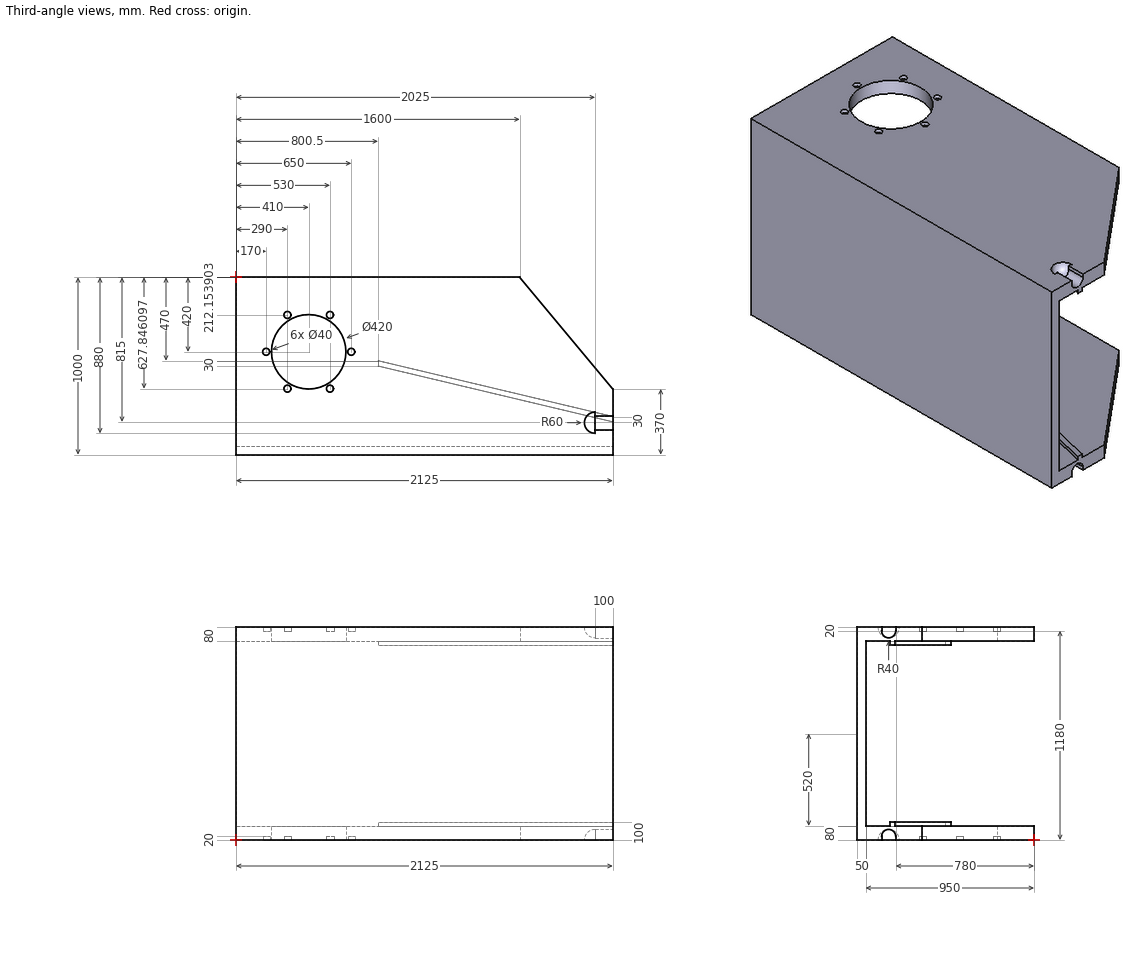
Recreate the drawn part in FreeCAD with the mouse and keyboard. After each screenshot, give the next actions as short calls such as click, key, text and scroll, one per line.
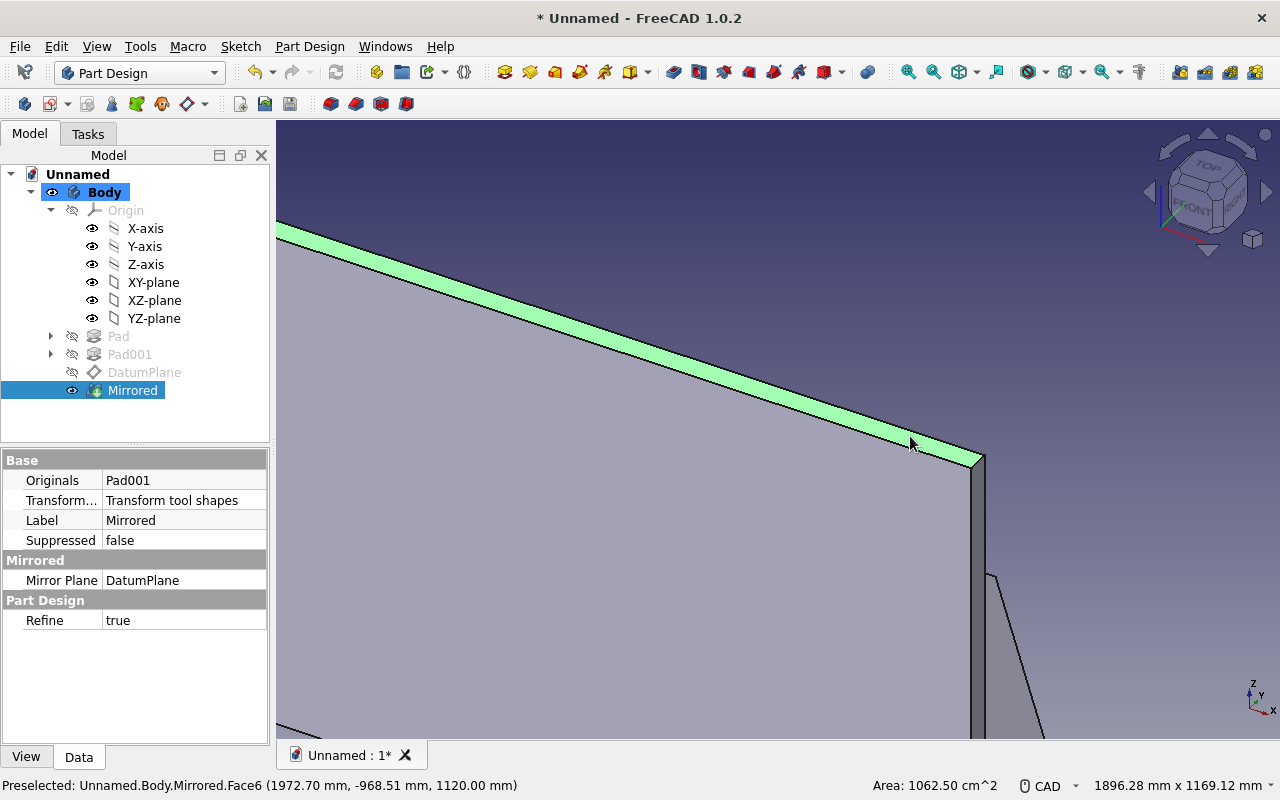
click(50, 104)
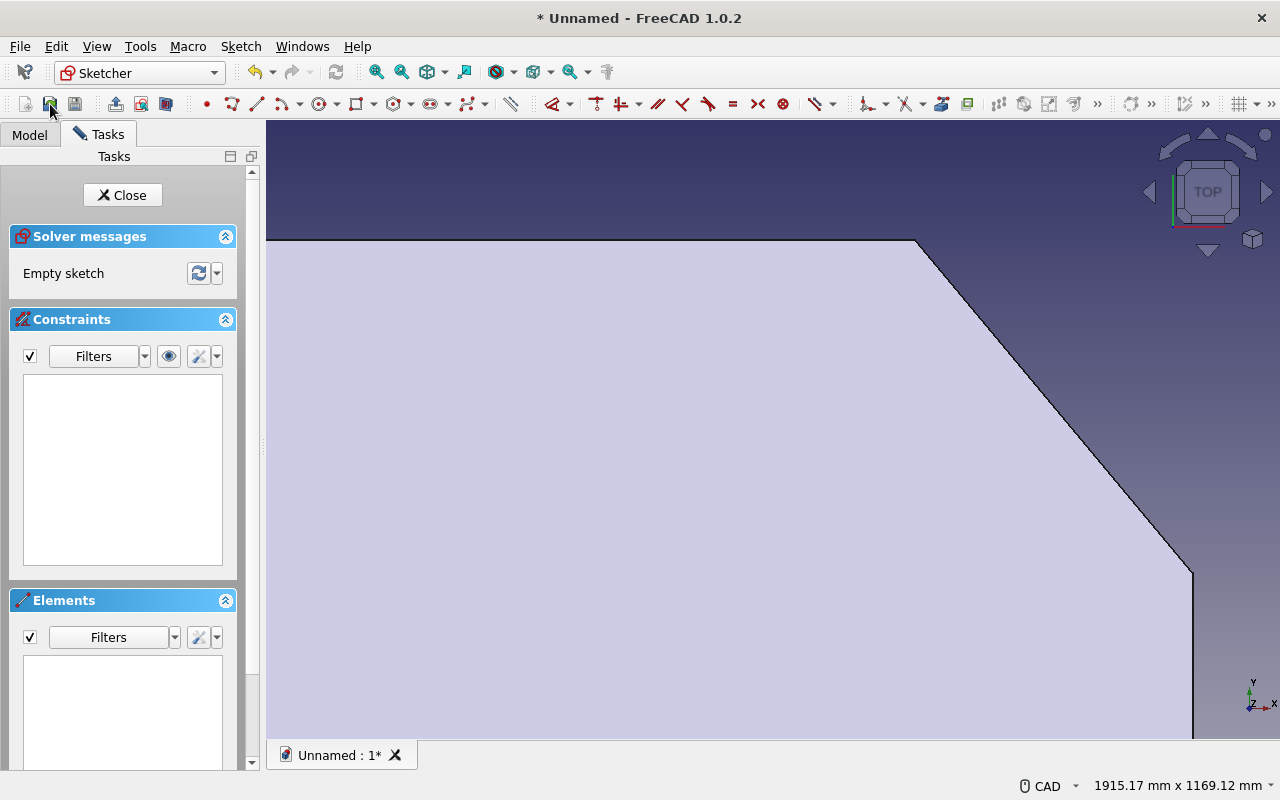
scroll(795, 338, down, 3)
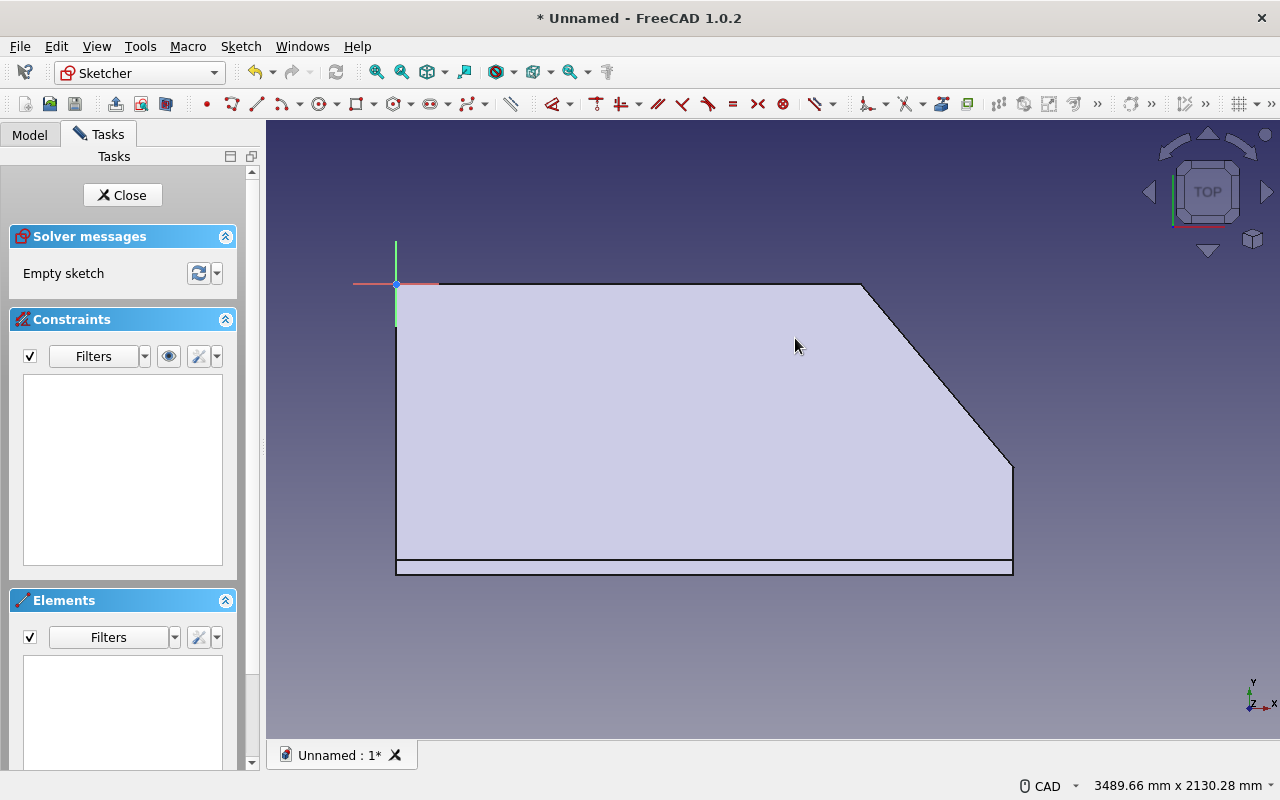
key(g)
key(m)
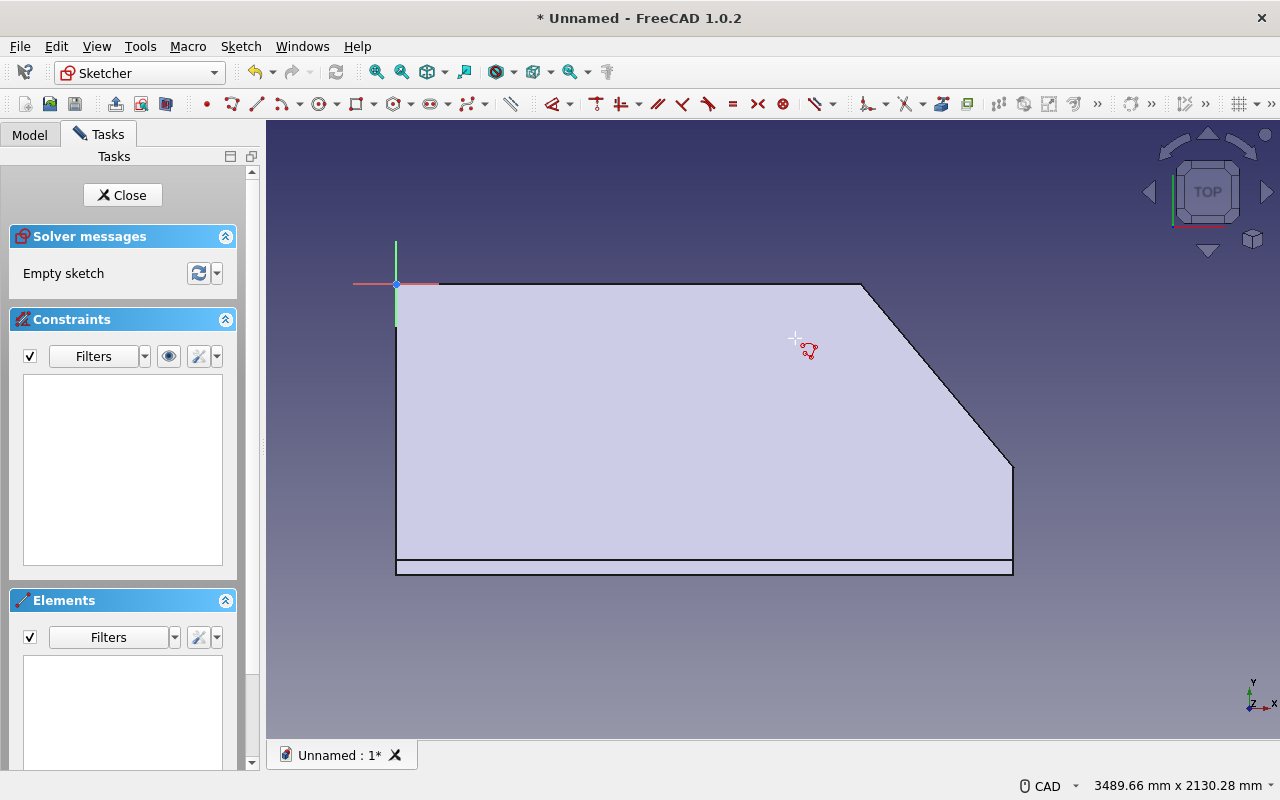
click(396, 284)
click(405, 575)
click(1013, 575)
click(1013, 467)
click(861, 293)
click(396, 284)
key(Escape)
key(Escape)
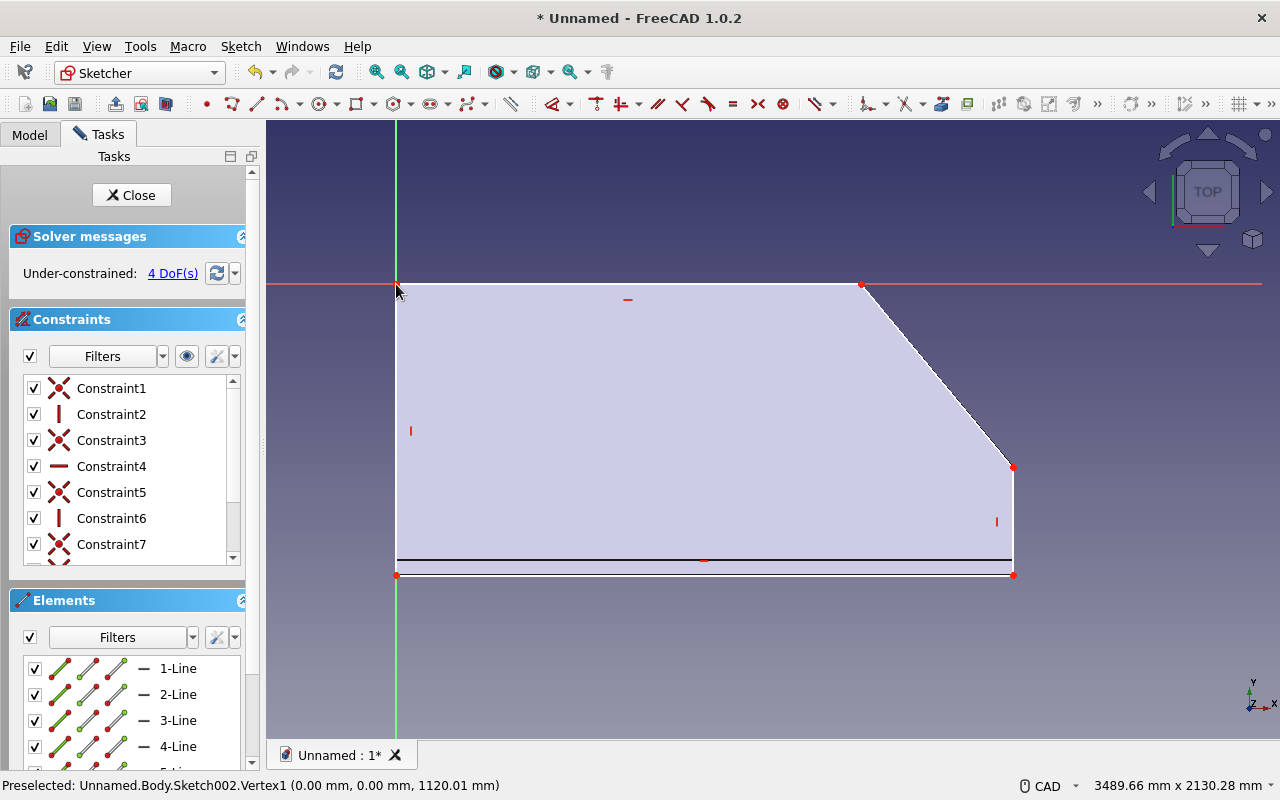
key(d)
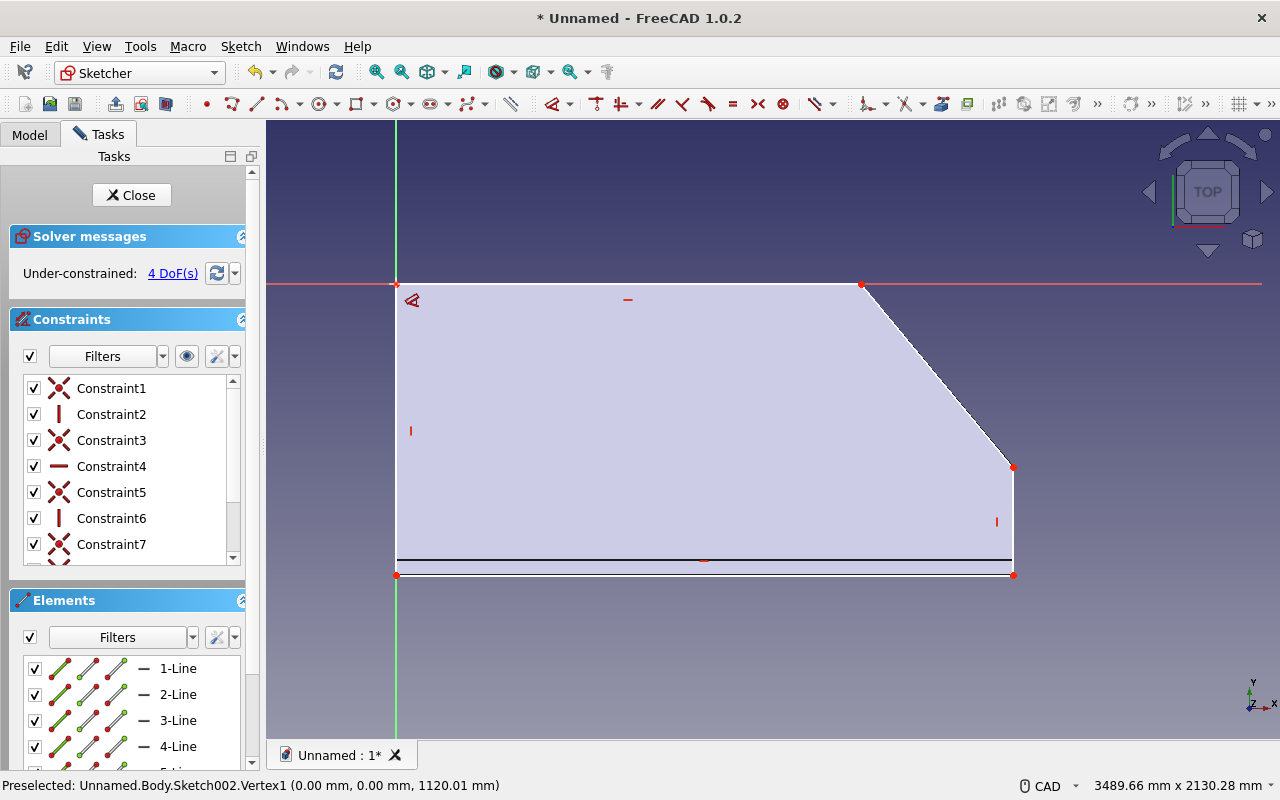
click(1013, 544)
click(1047, 522)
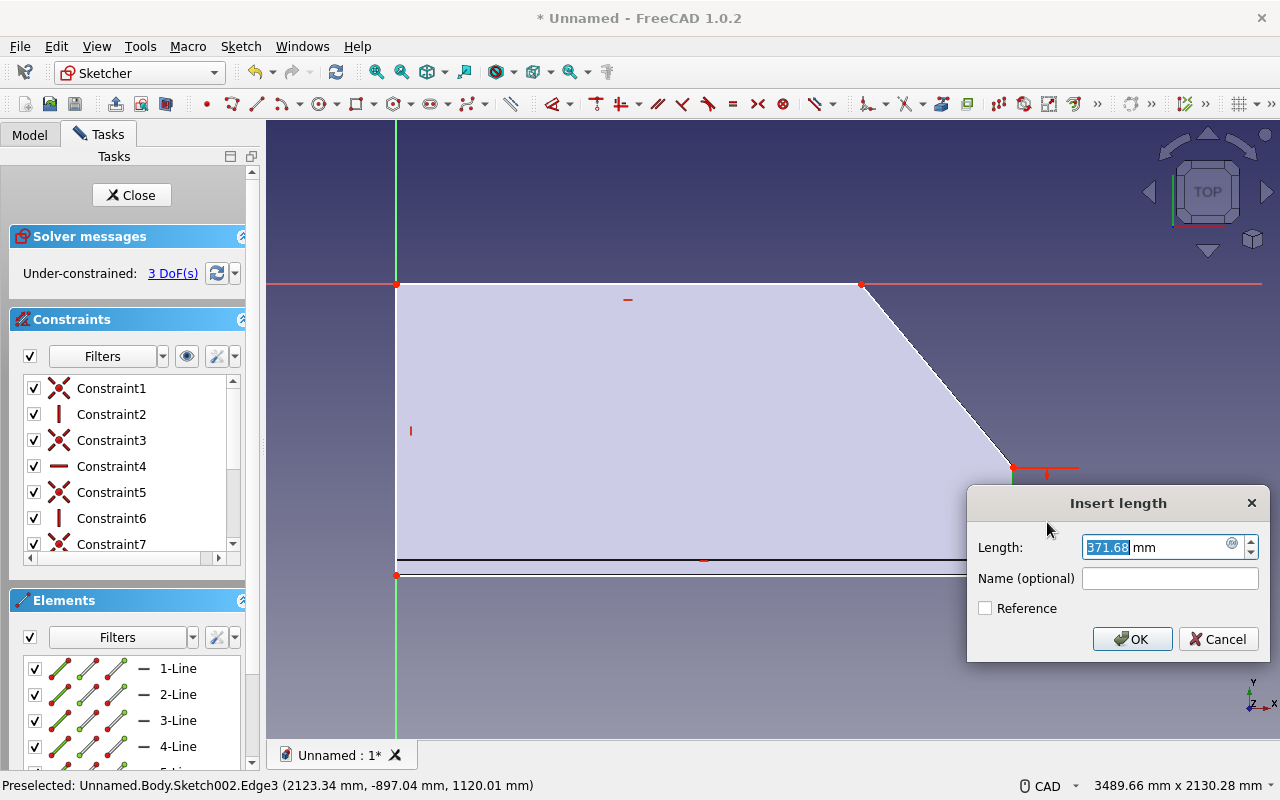
text(370)
key(Return)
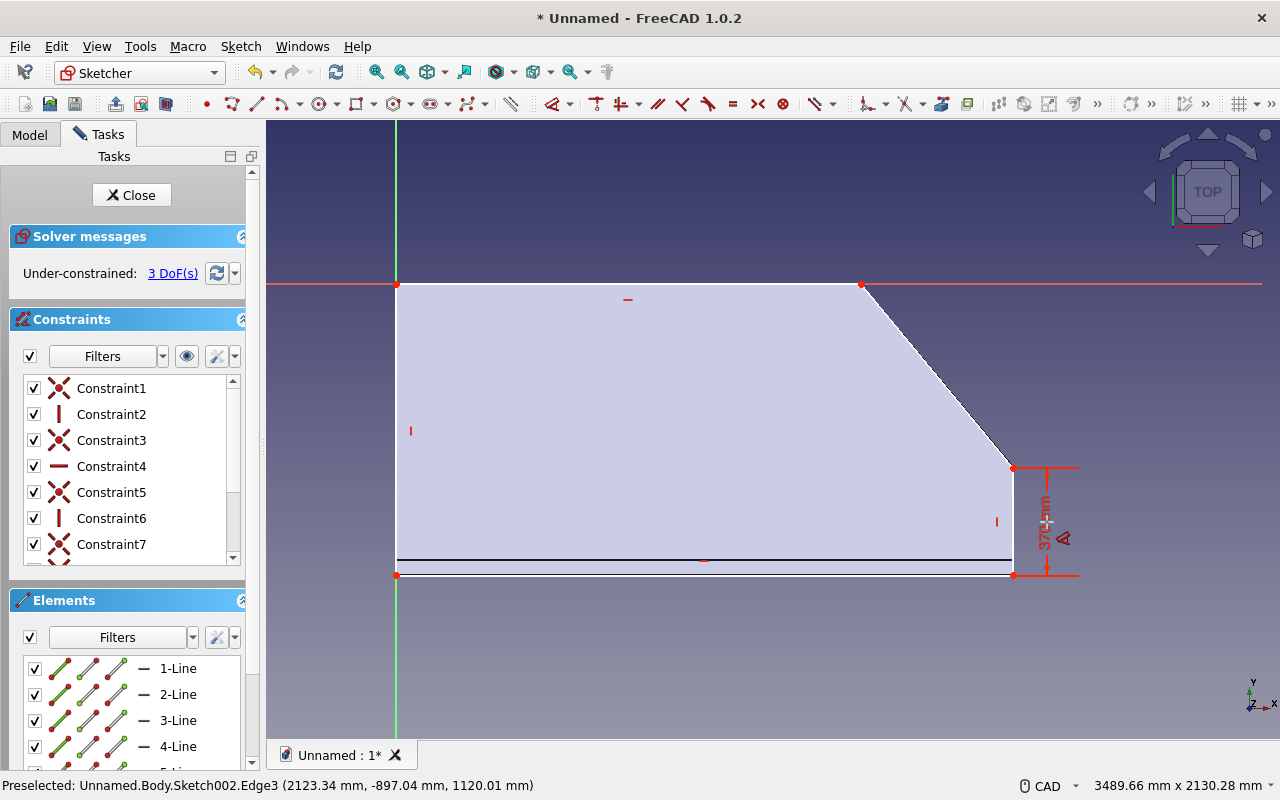
click(396, 372)
click(362, 430)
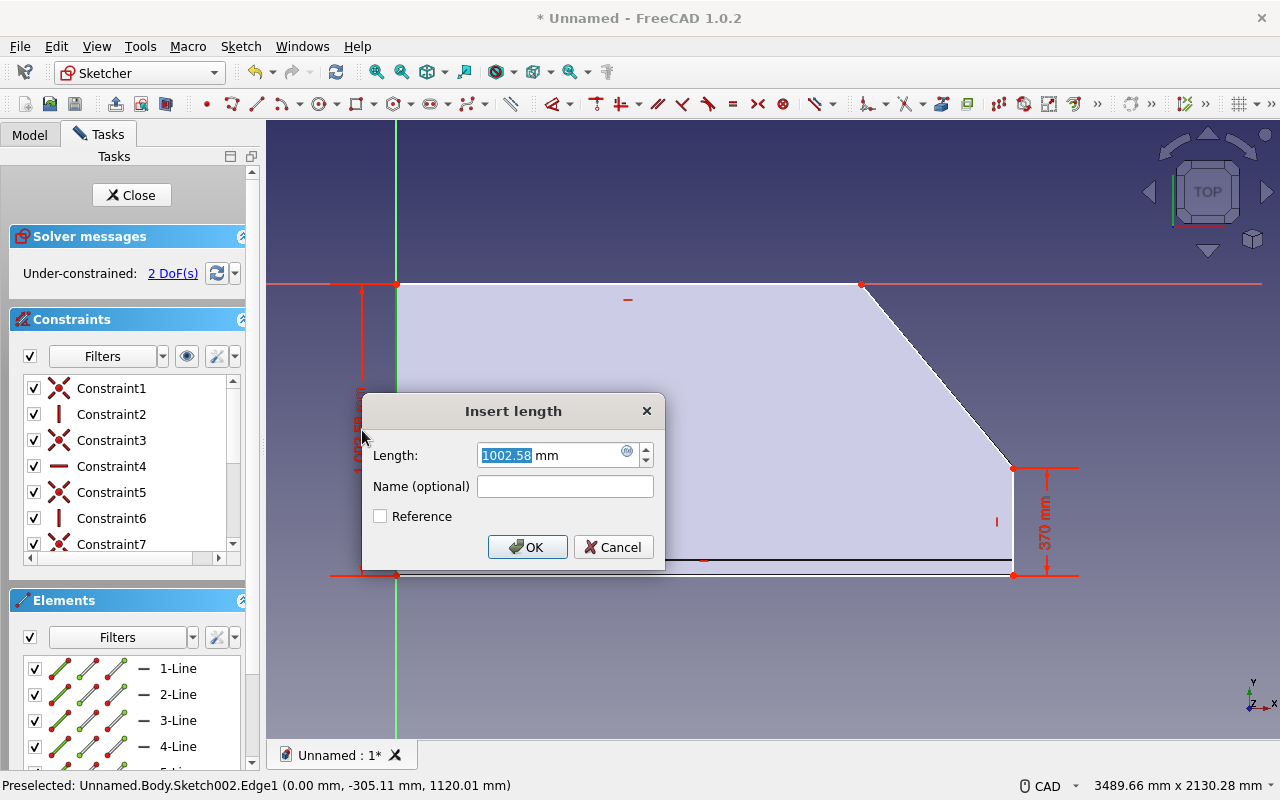
text(1000)
key(Return)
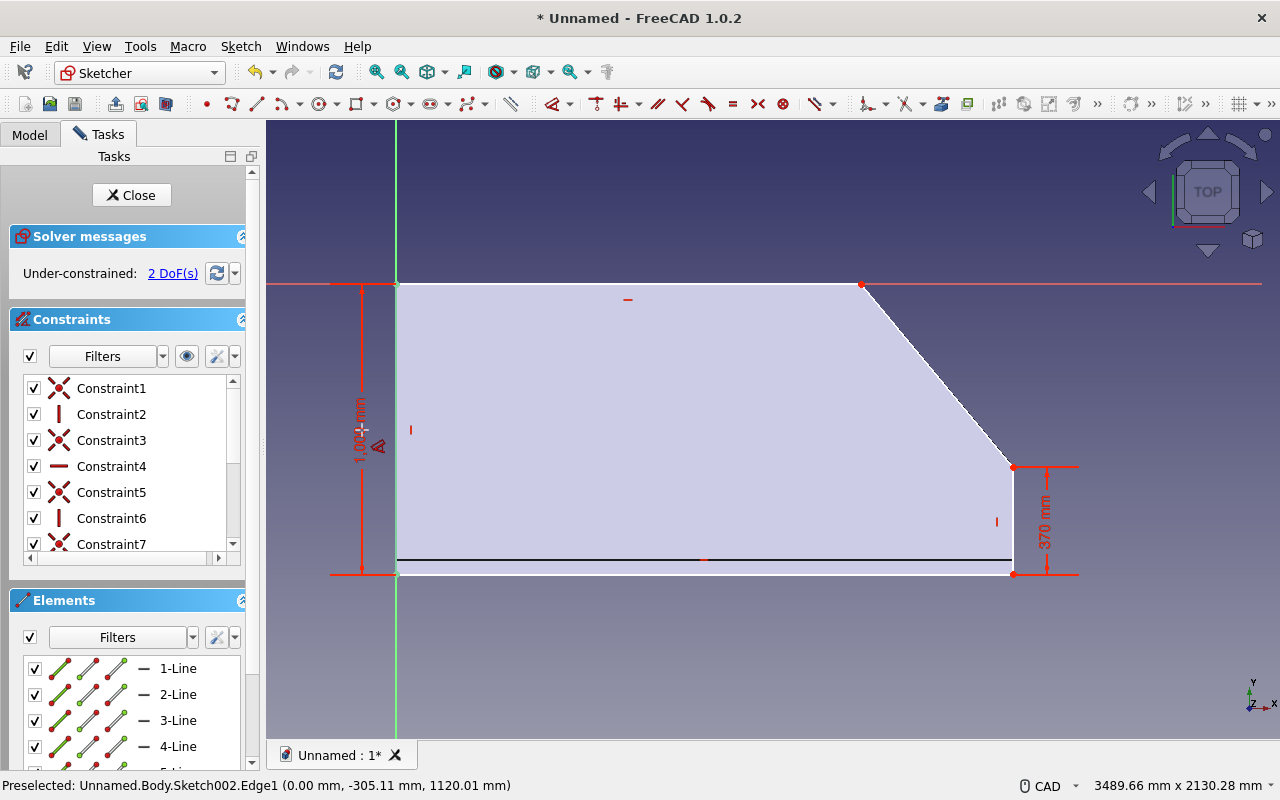
click(581, 575)
click(705, 609)